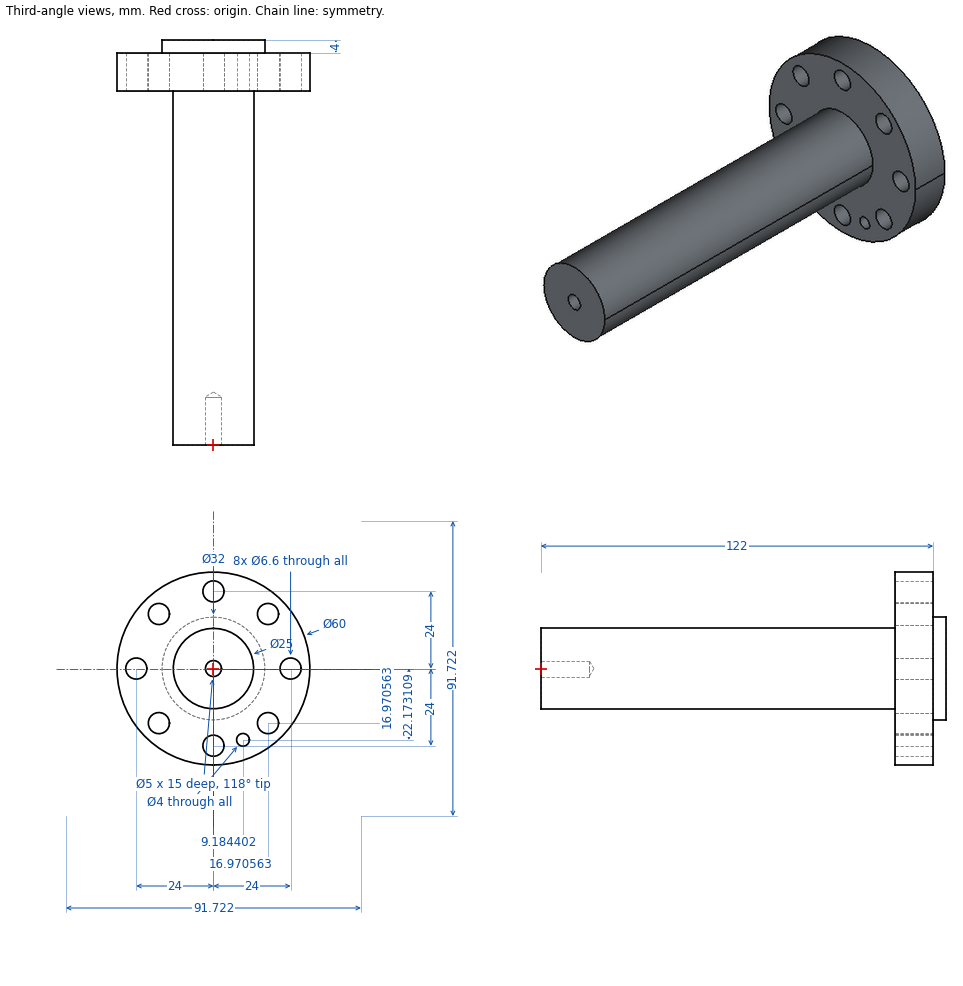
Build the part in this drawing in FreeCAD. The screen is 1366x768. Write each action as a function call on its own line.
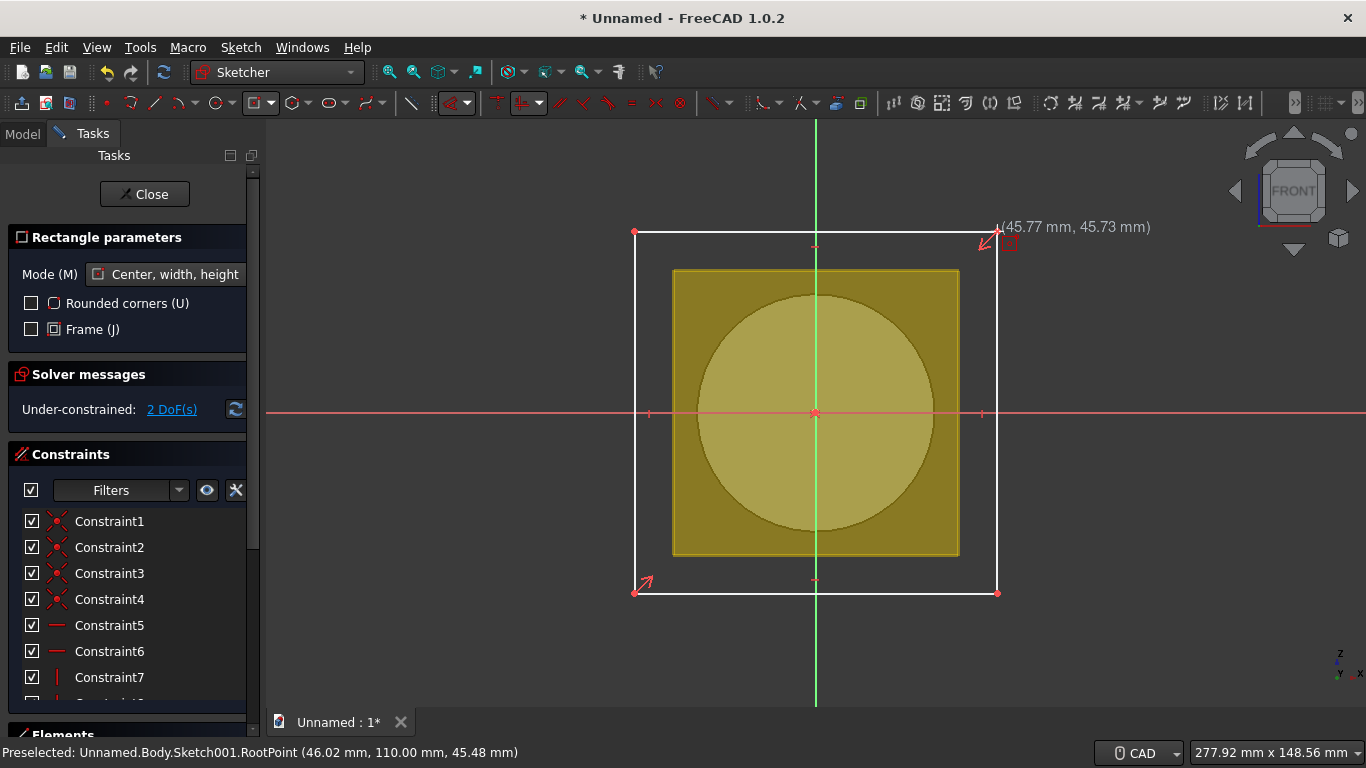
click(216, 104)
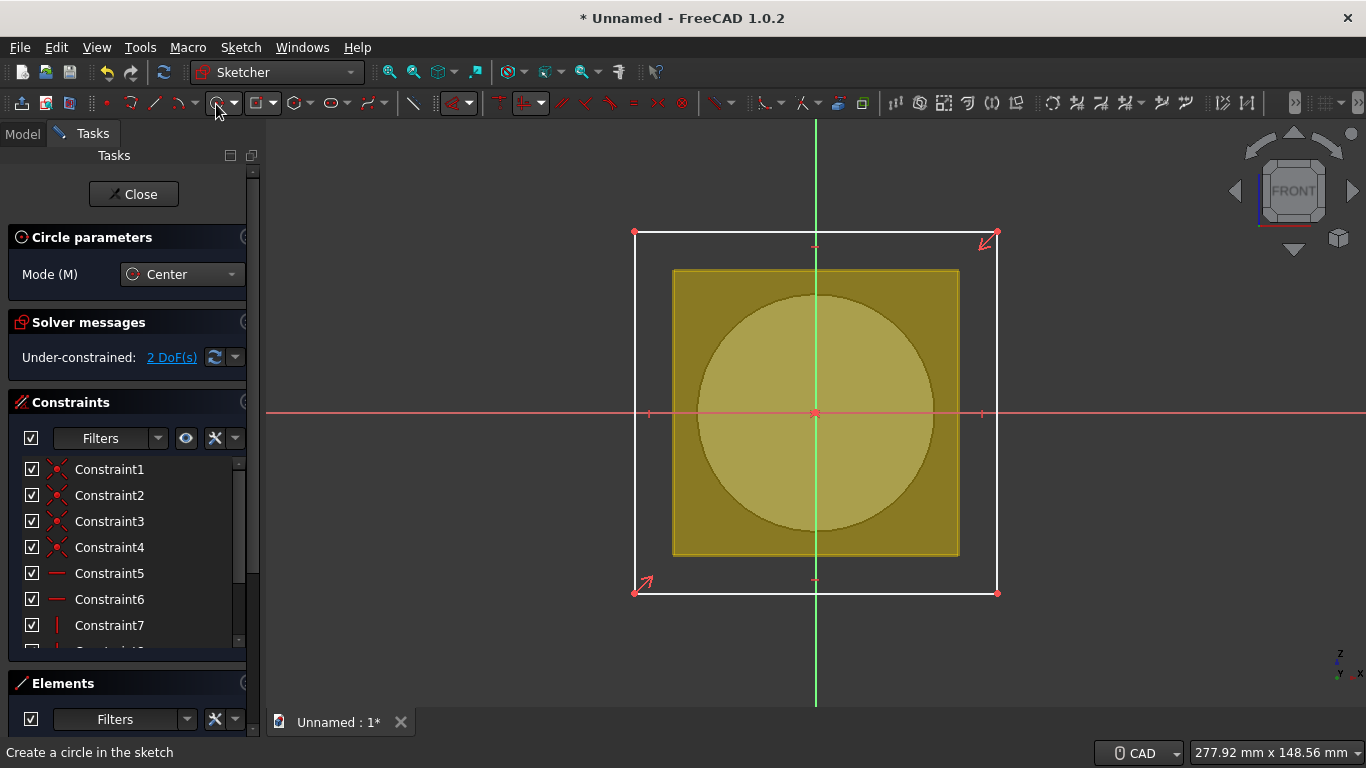
click(816, 413)
click(851, 378)
key(Escape)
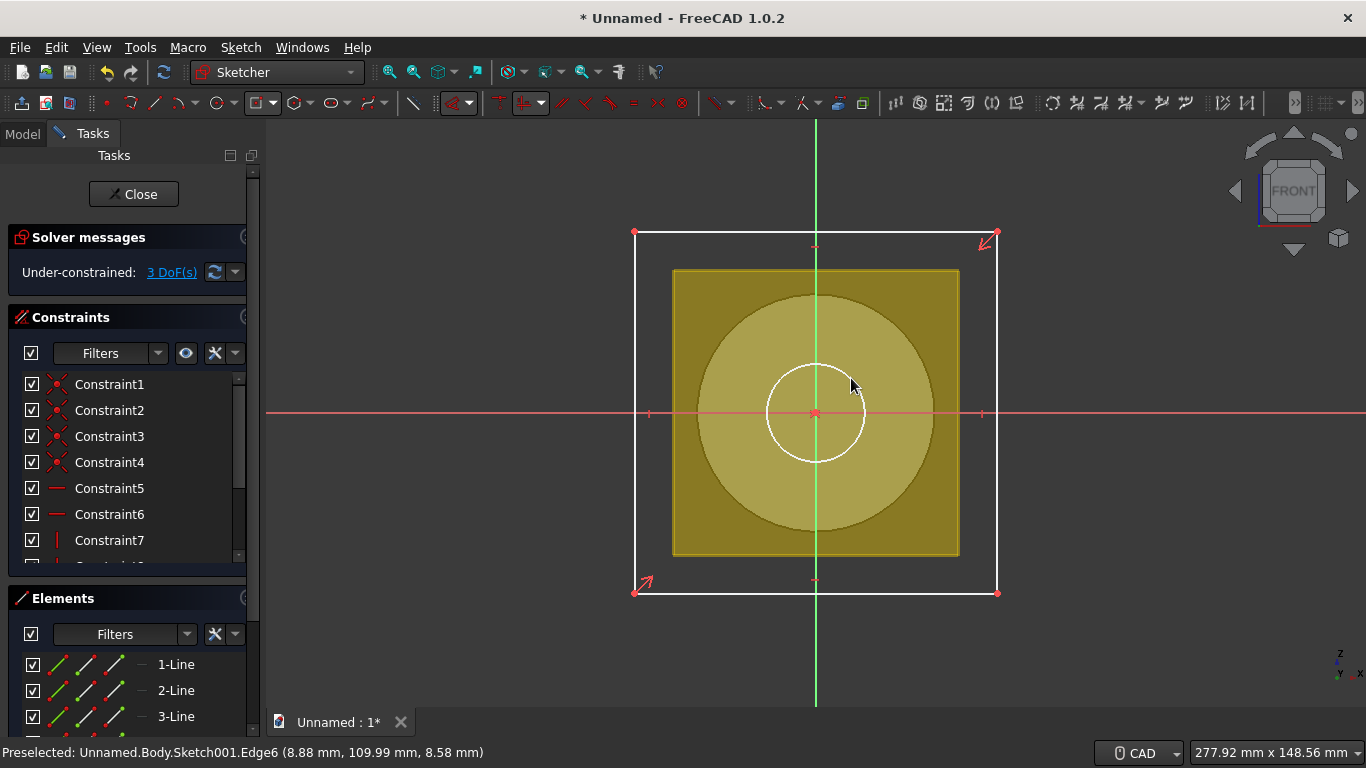
click(850, 378)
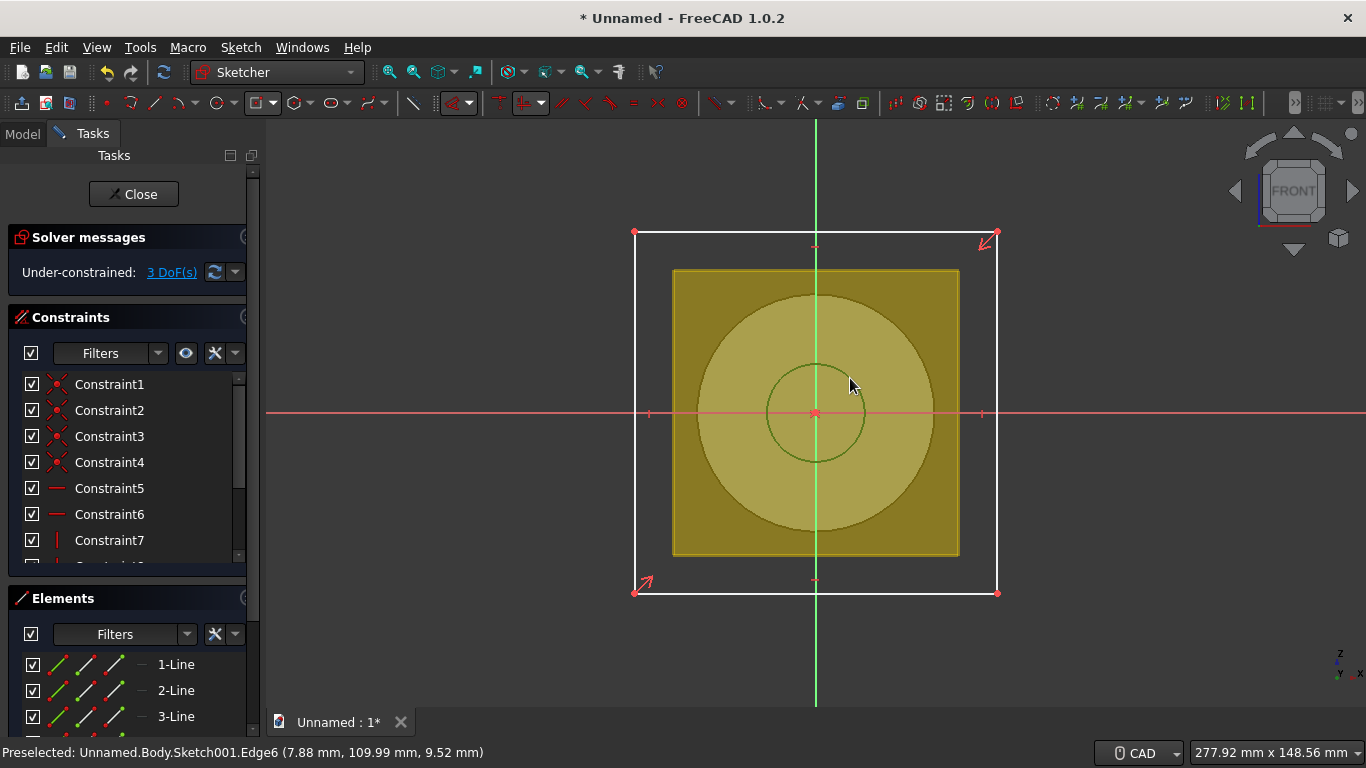
key(k)
key(o)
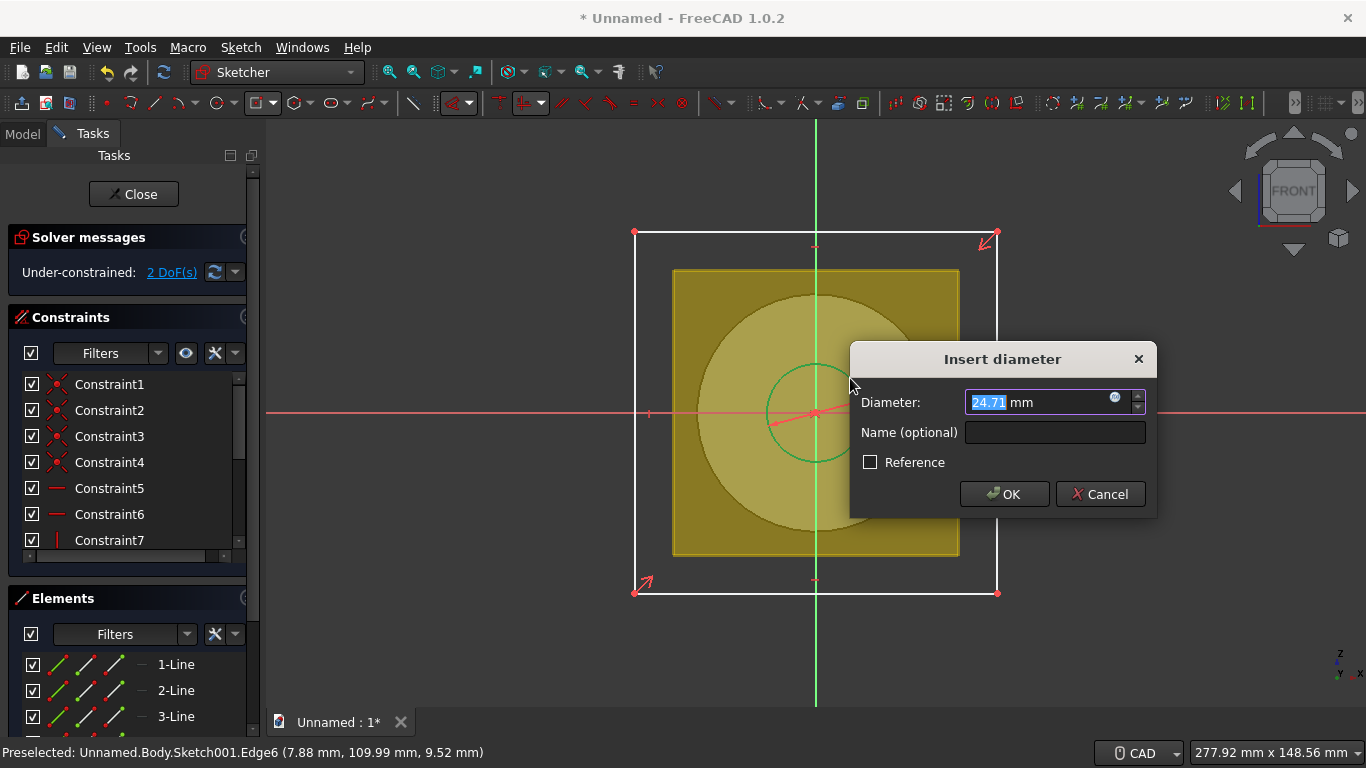
text(25)
key(Return)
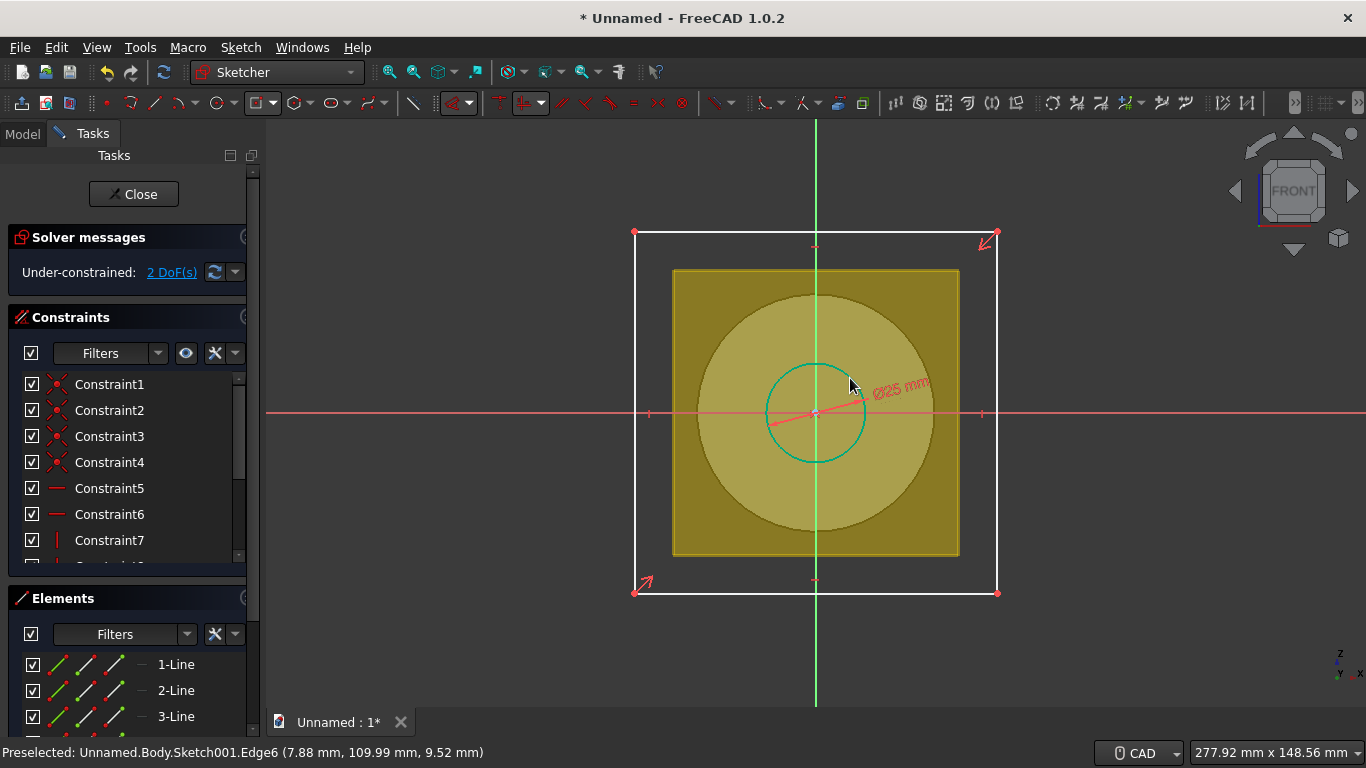
click(743, 594)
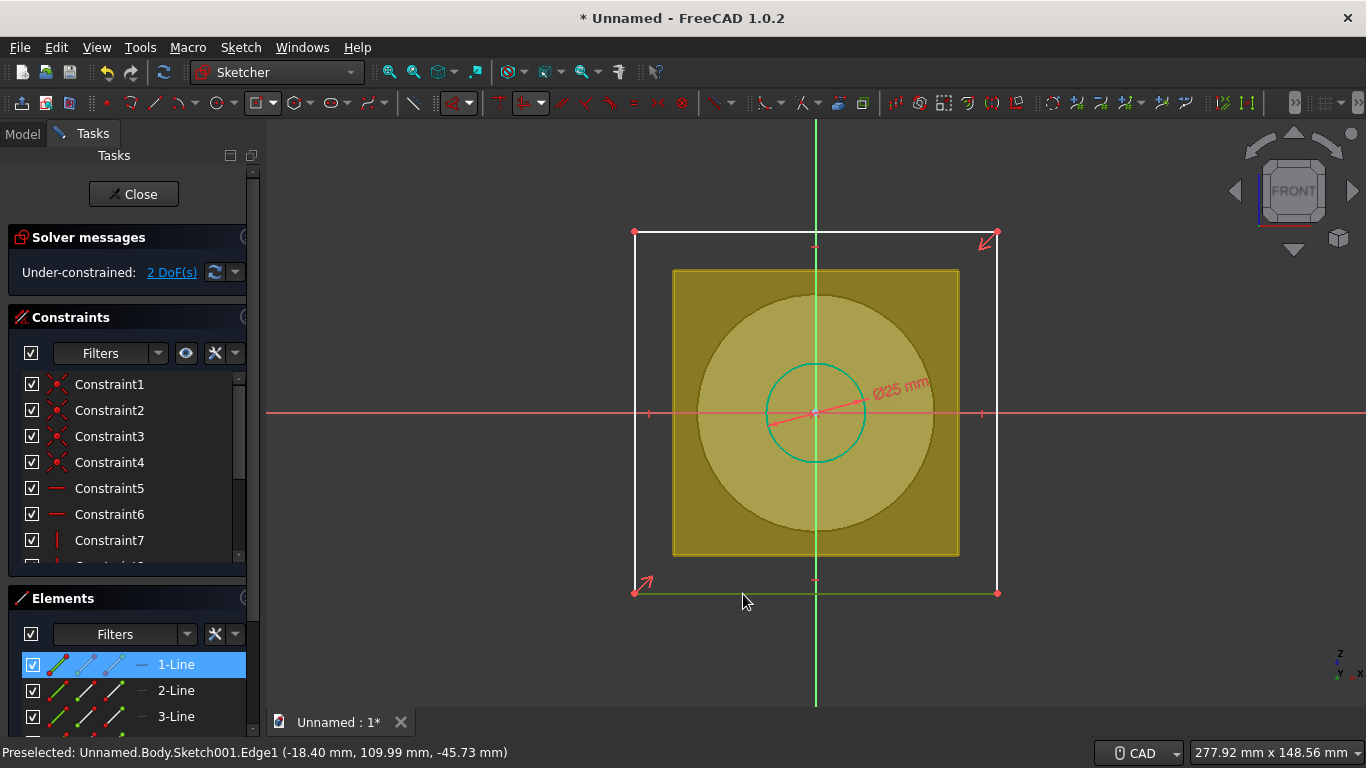
click(472, 104)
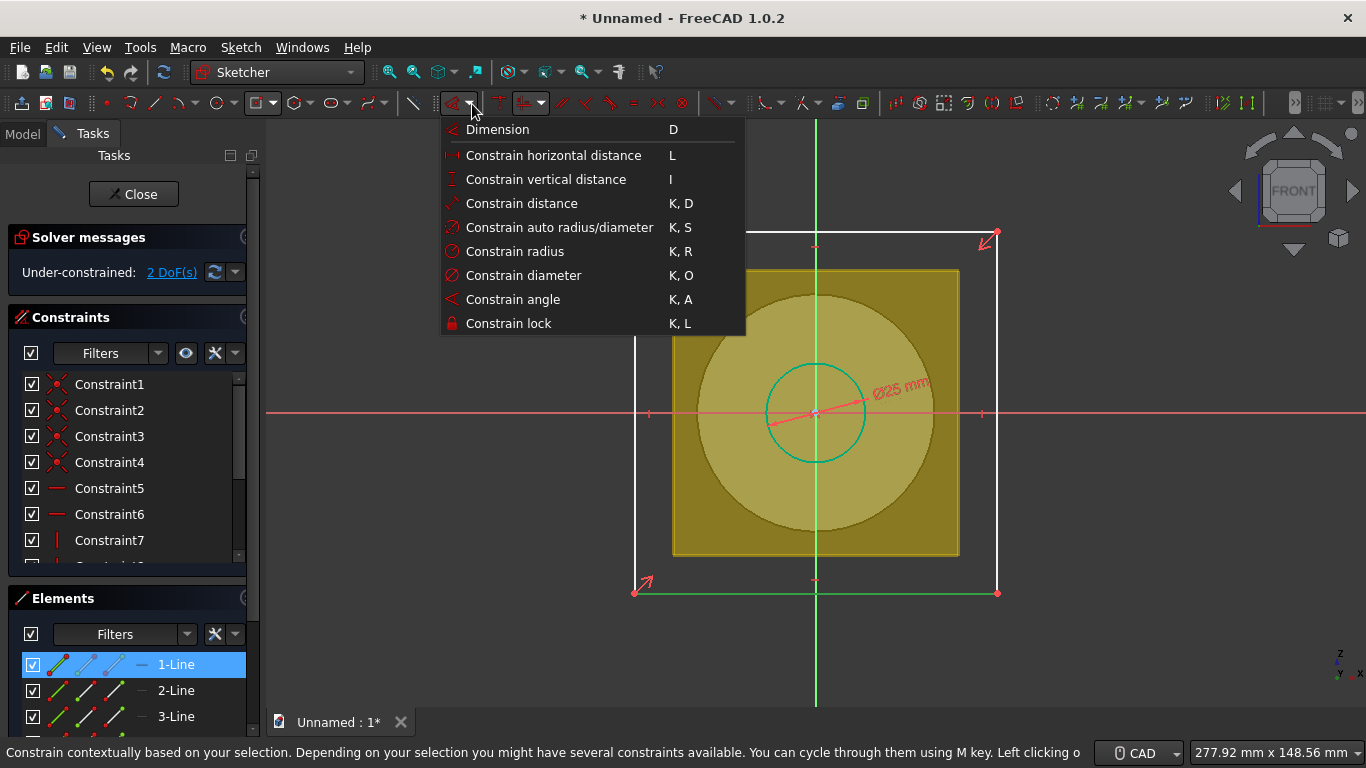
click(593, 155)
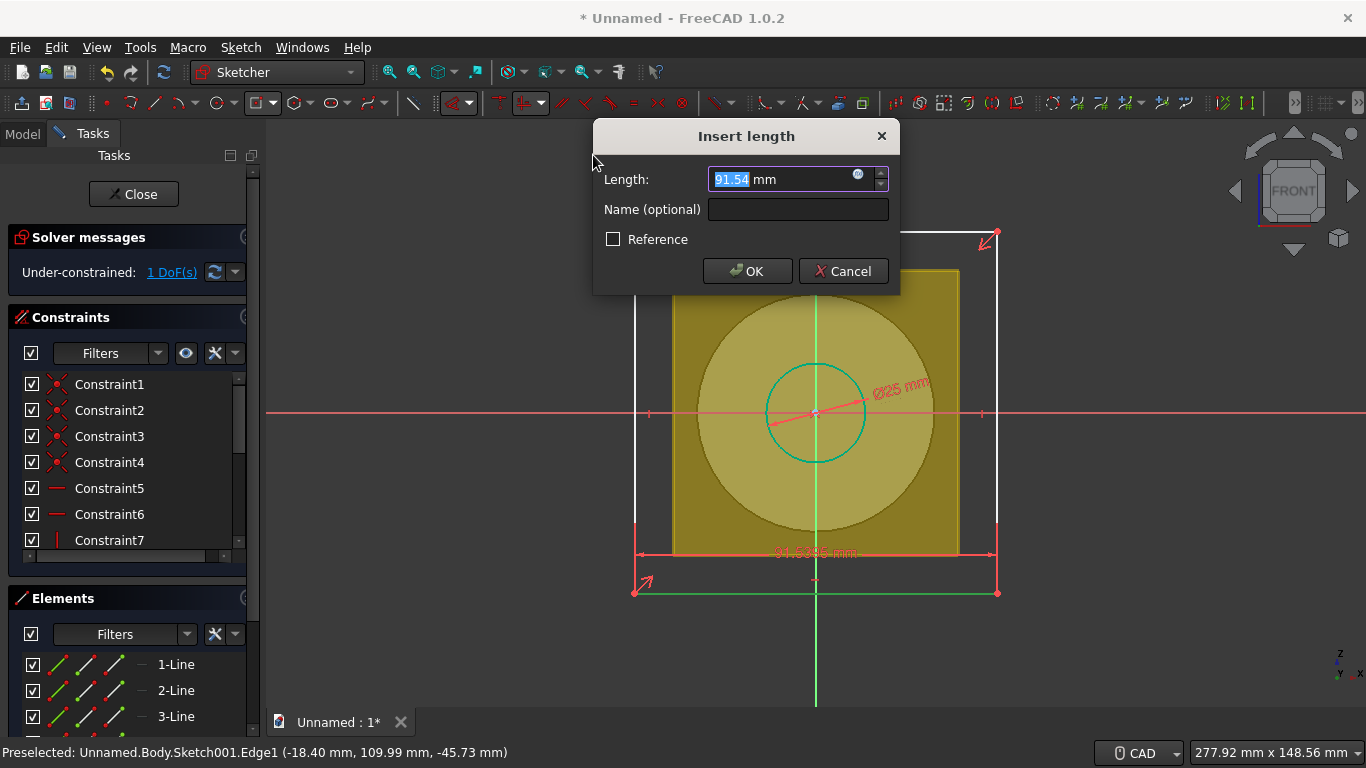
text(91.722)
key(Return)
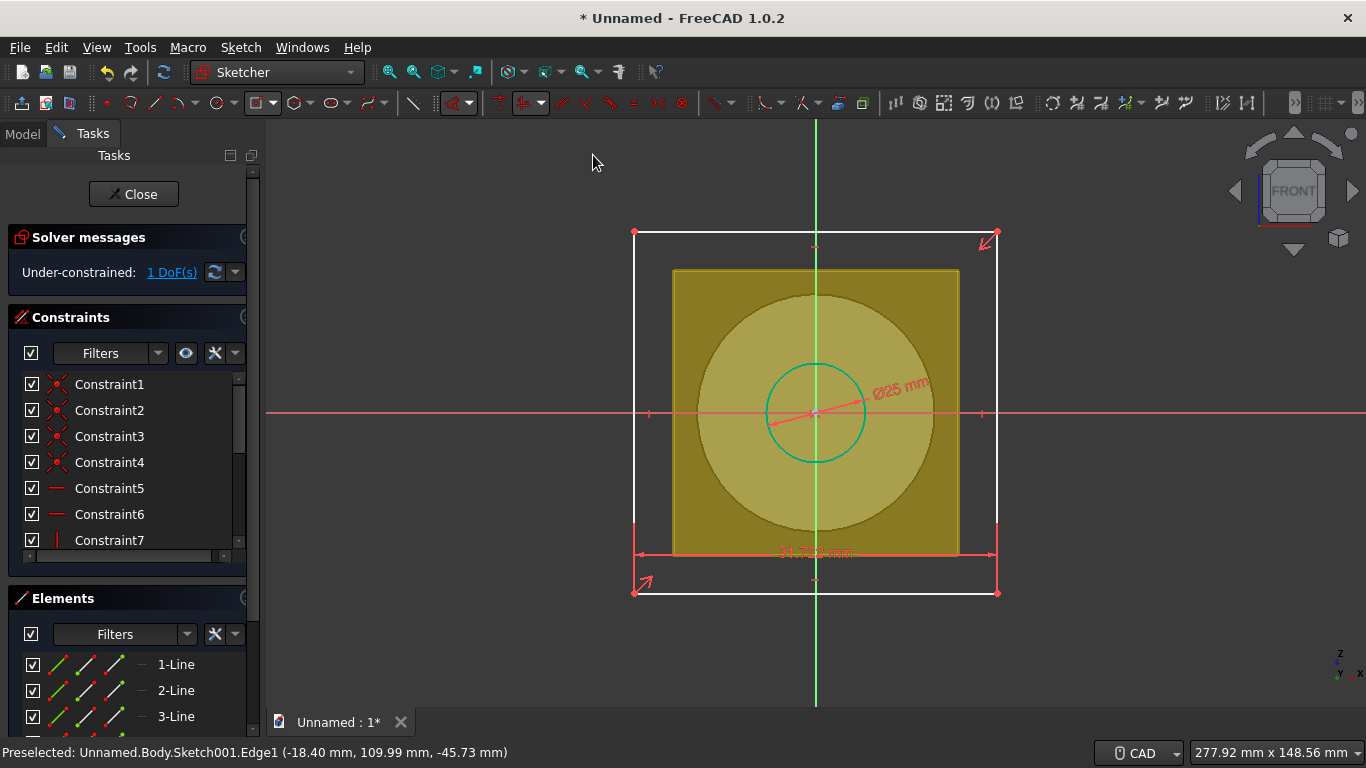
click(997, 485)